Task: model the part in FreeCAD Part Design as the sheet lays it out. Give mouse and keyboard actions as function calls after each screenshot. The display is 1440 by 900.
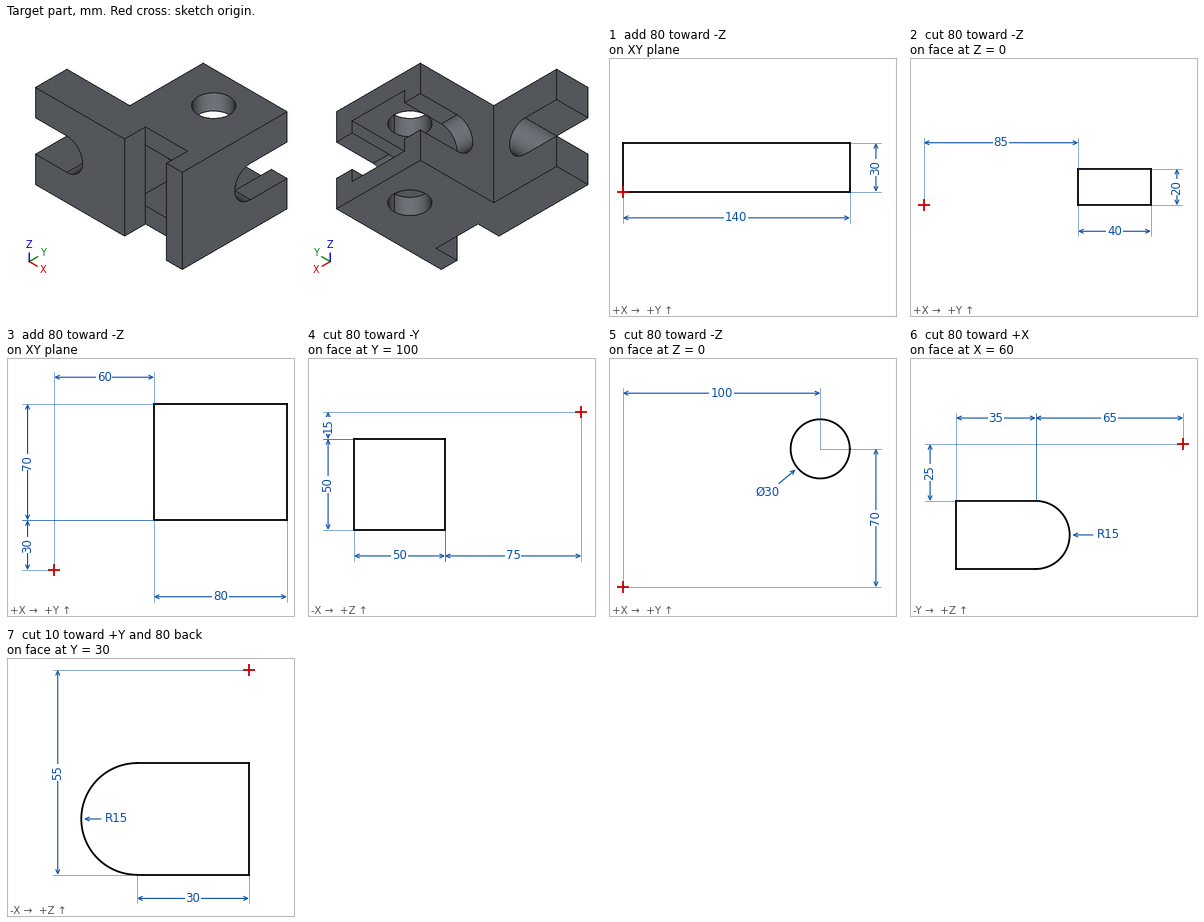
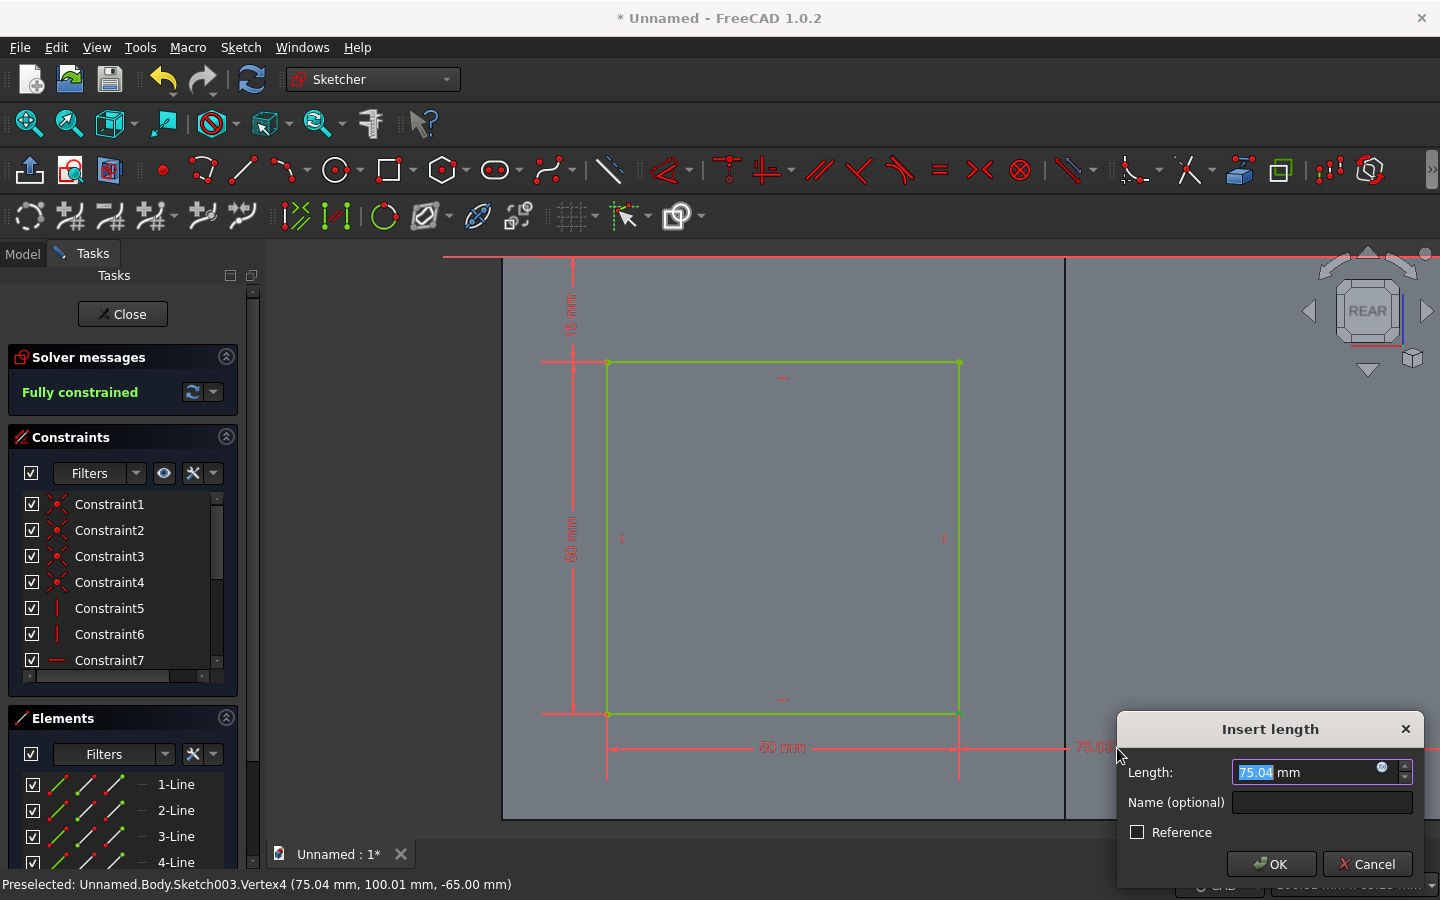
text(75)
key(Return)
key(Escape)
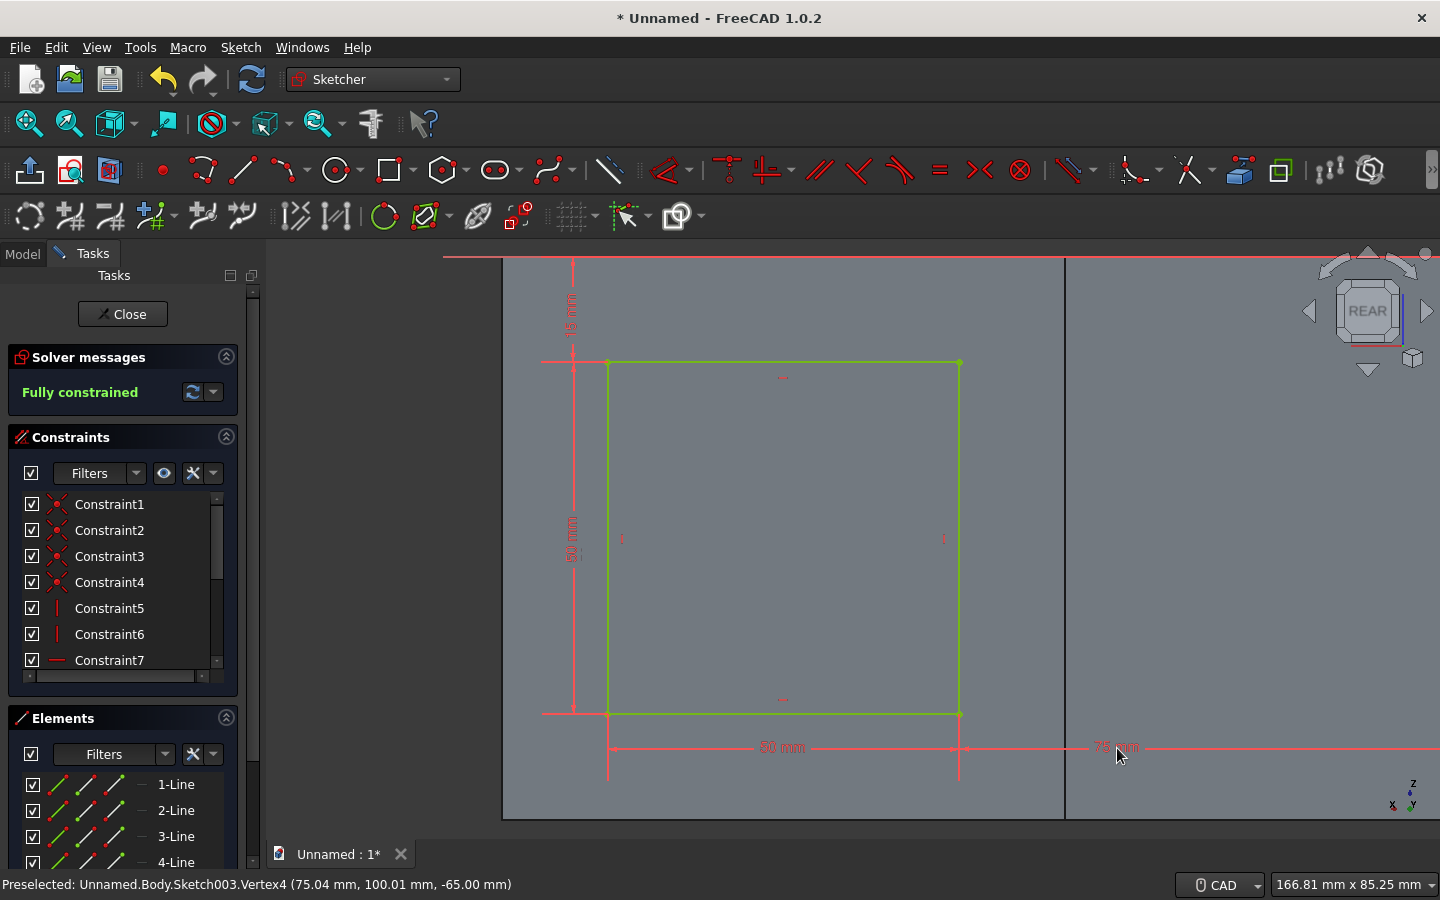
click(123, 314)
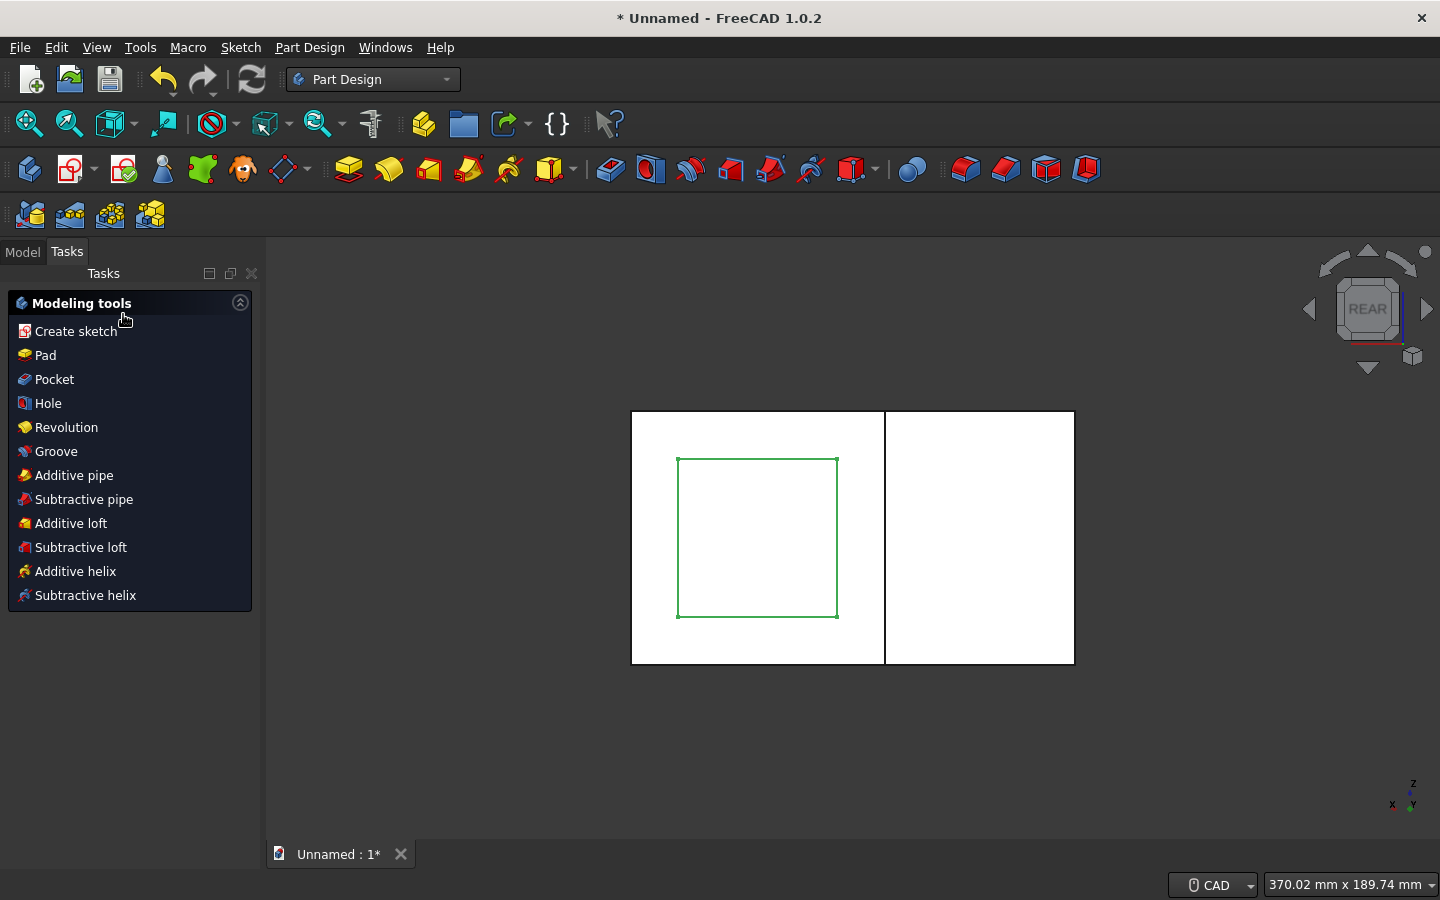
click(612, 170)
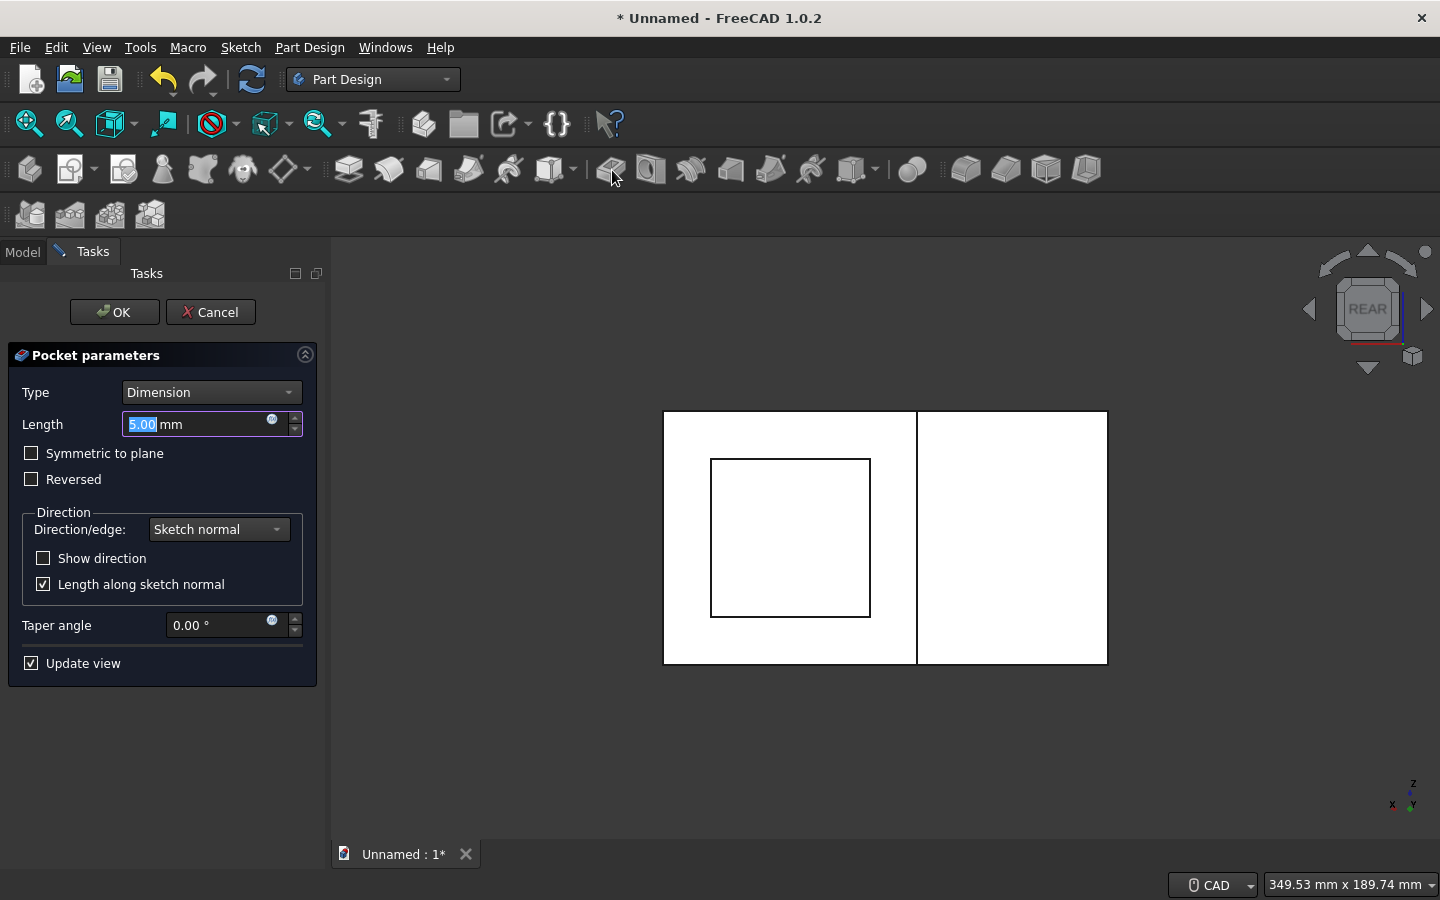
text(80)
key(Tab)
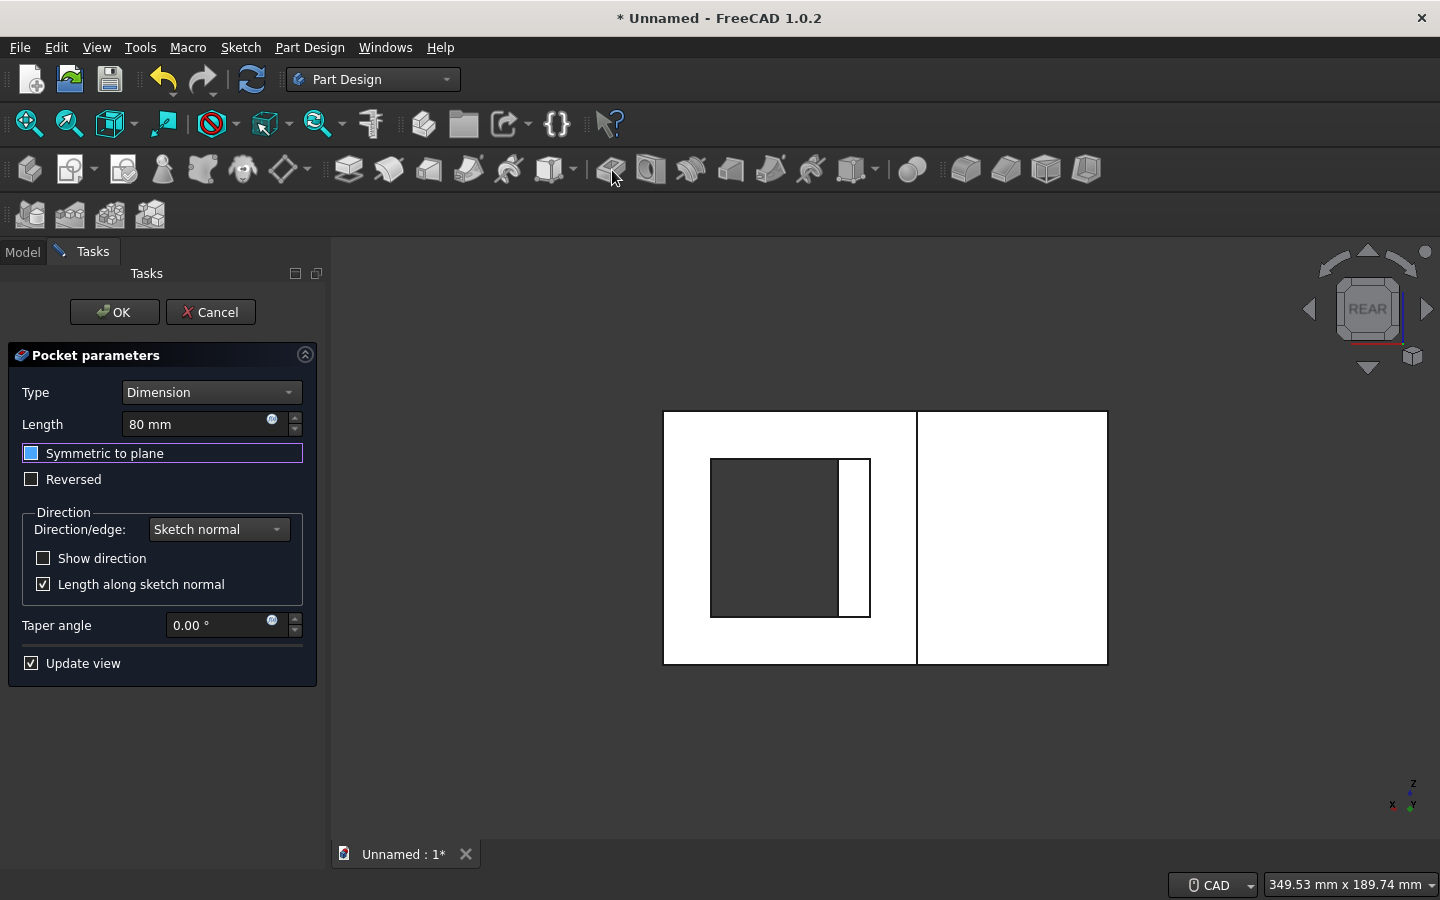
click(115, 312)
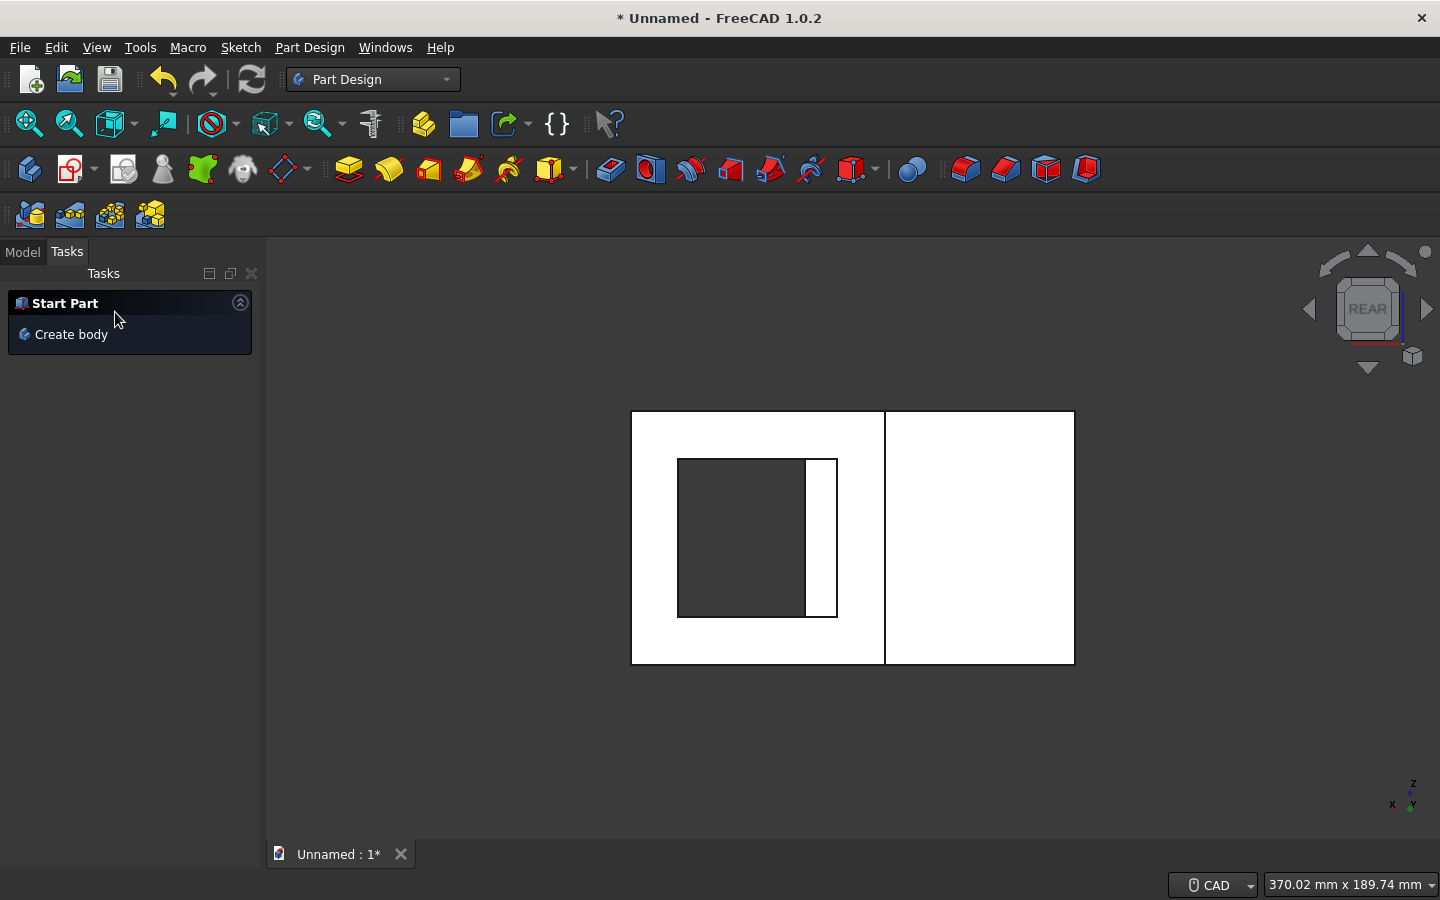
click(30, 124)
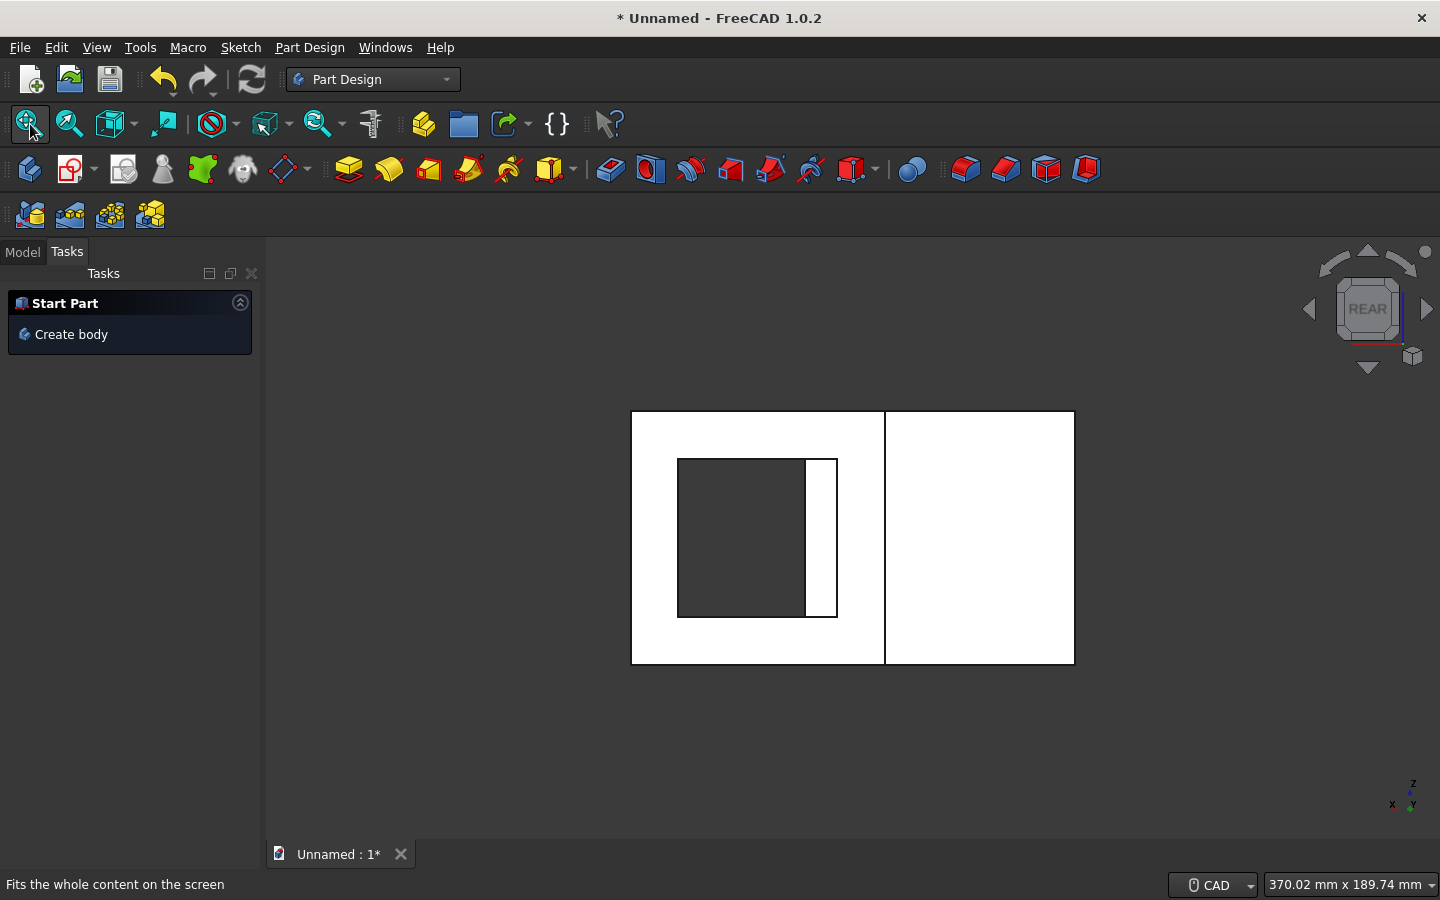
key(0)